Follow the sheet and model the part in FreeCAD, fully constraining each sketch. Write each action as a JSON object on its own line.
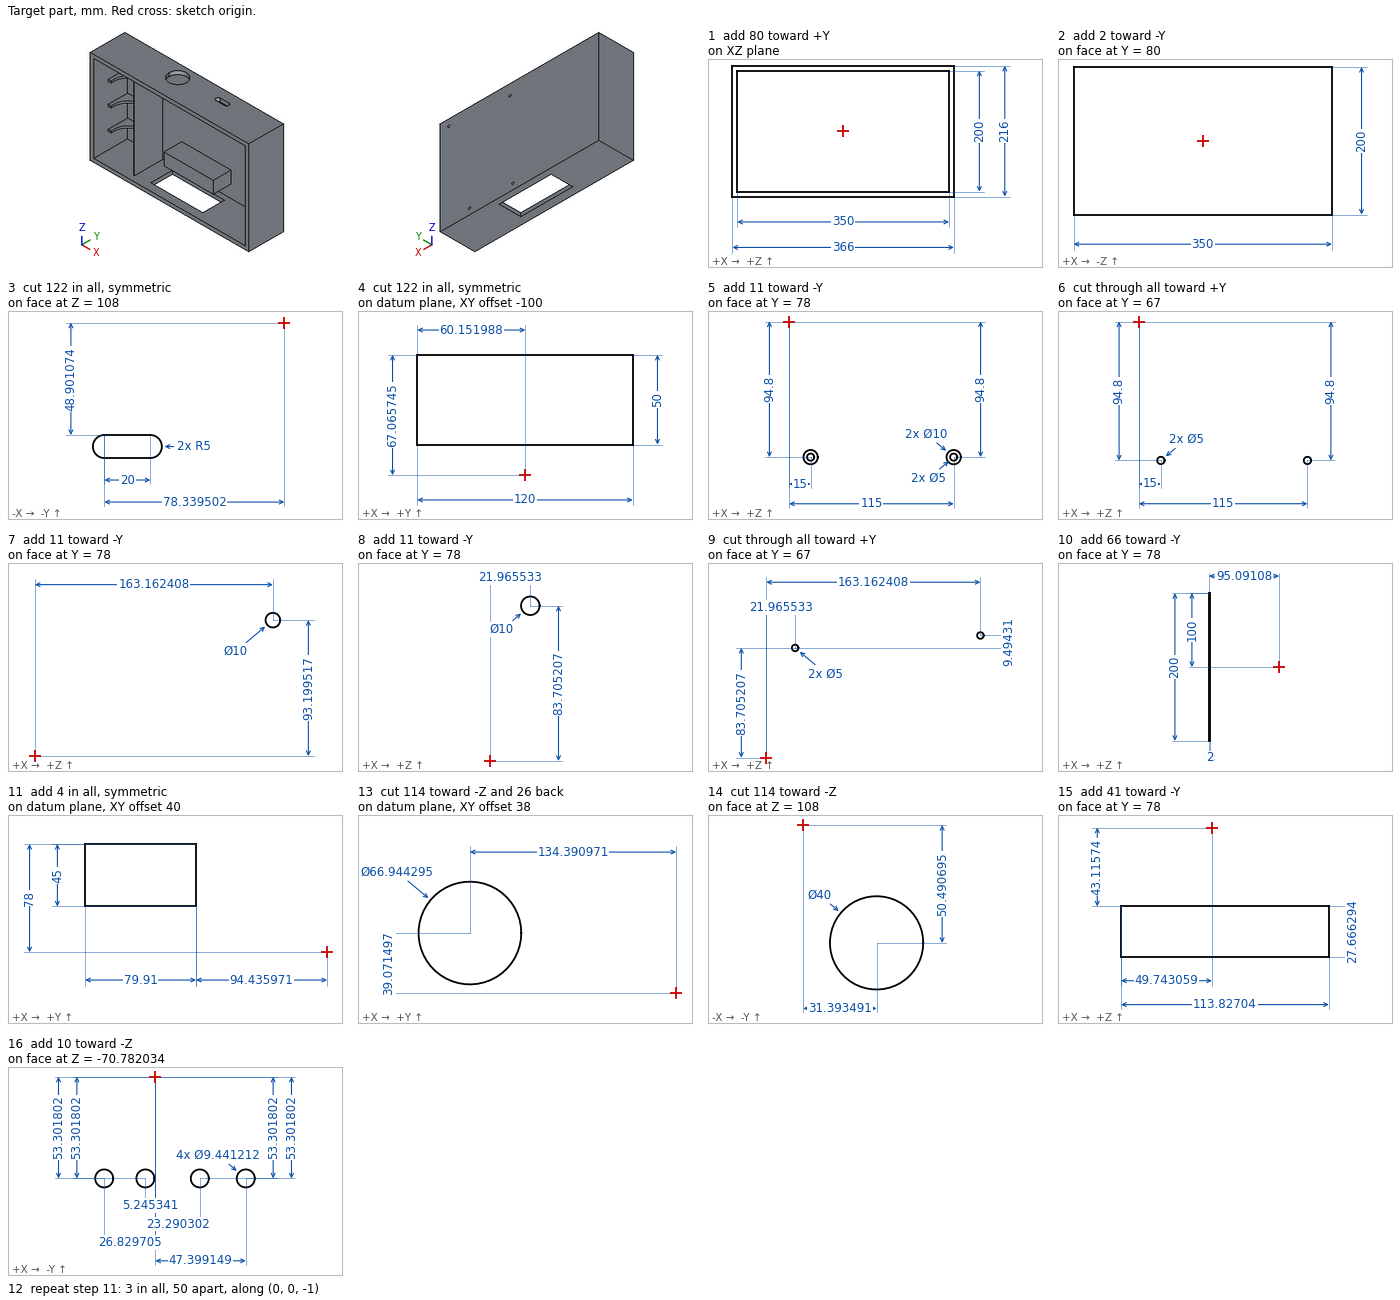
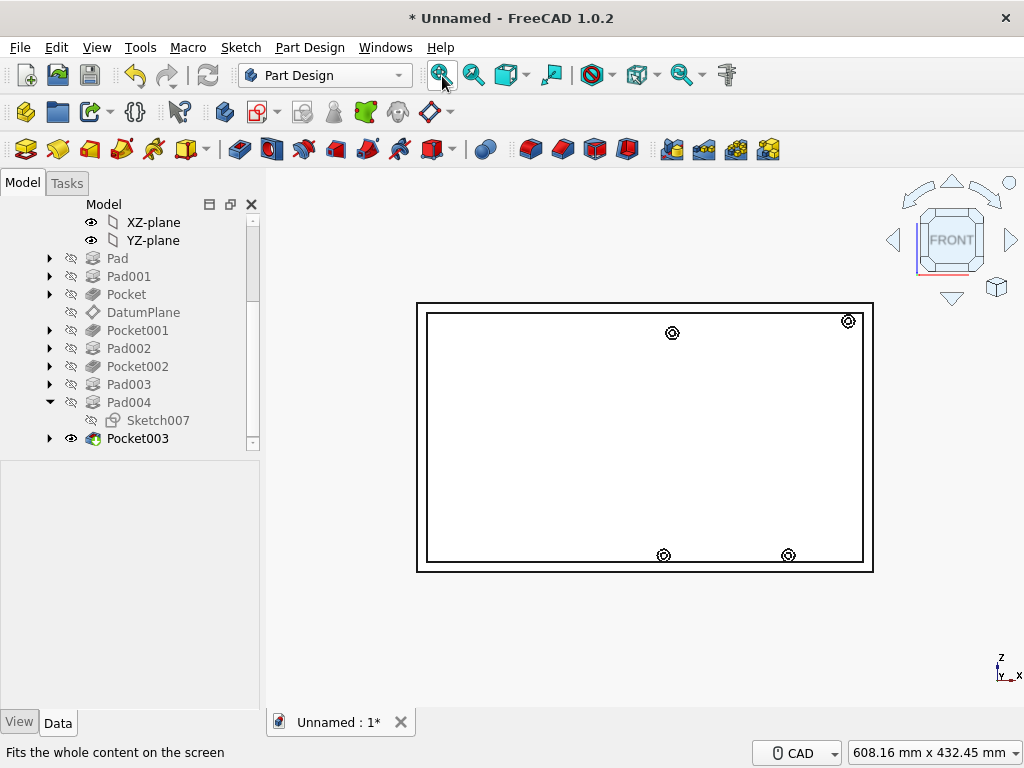
{"action": "left_click", "coordinate": [583, 437]}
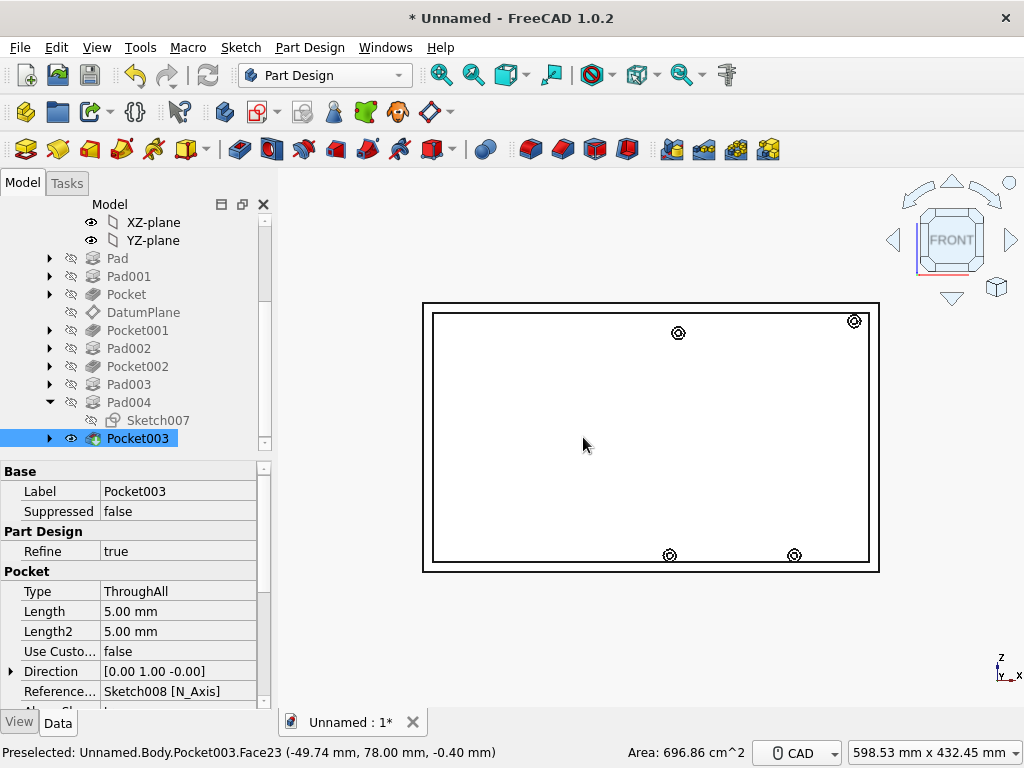
{"action": "left_click", "coordinate": [258, 112]}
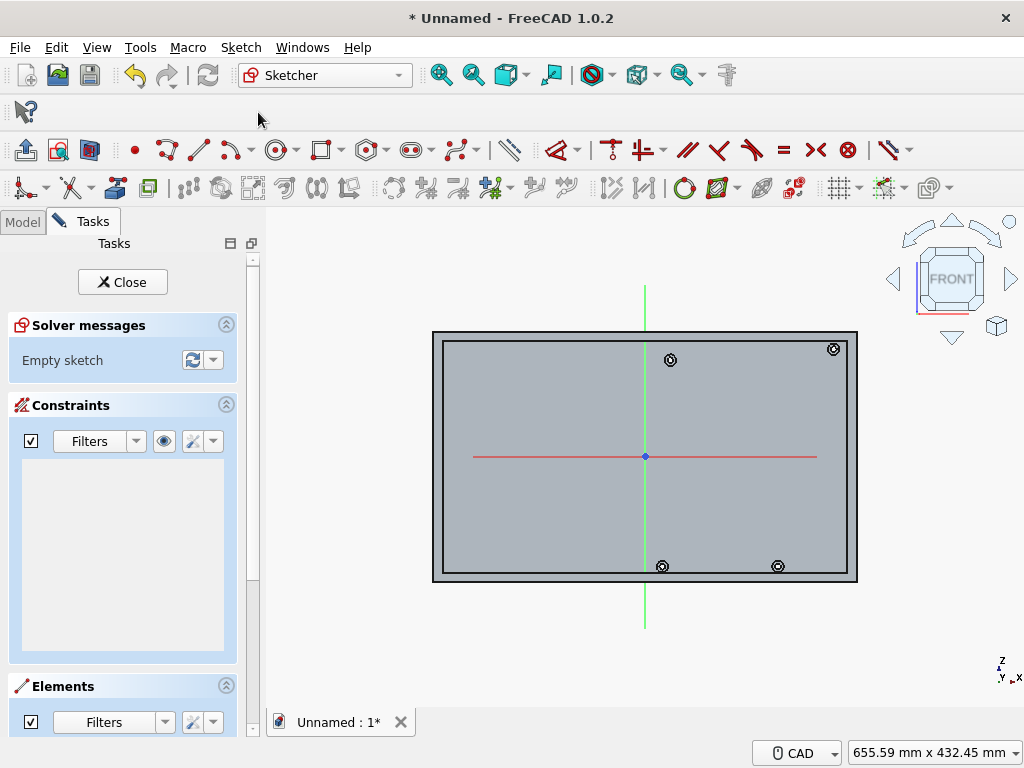
{"action": "scroll", "coordinate": [618, 457], "scroll_direction": "up", "scroll_amount": 2}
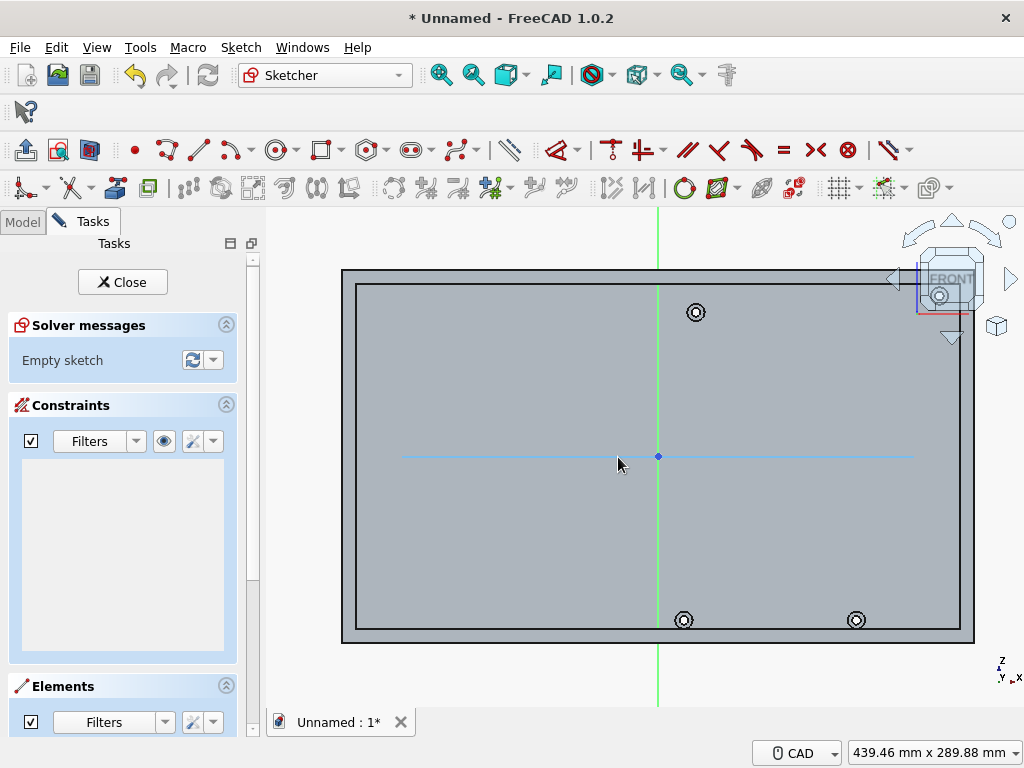
{"action": "key", "text": "g r"}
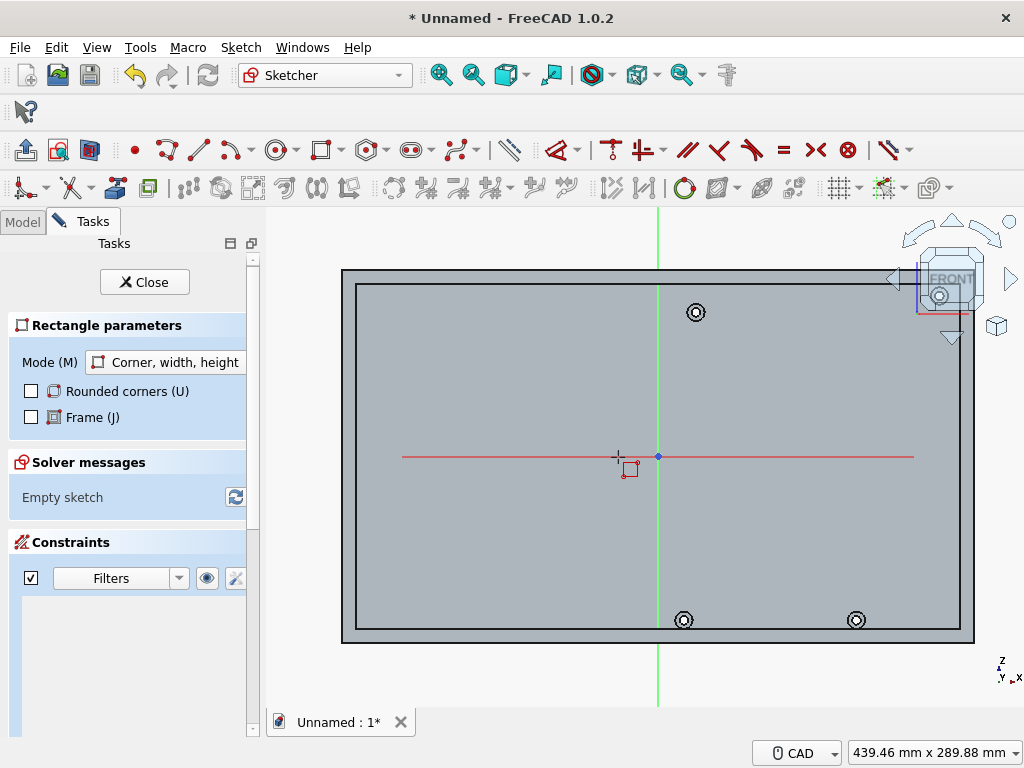
{"action": "scroll", "coordinate": [494, 284], "scroll_direction": "up", "scroll_amount": 8}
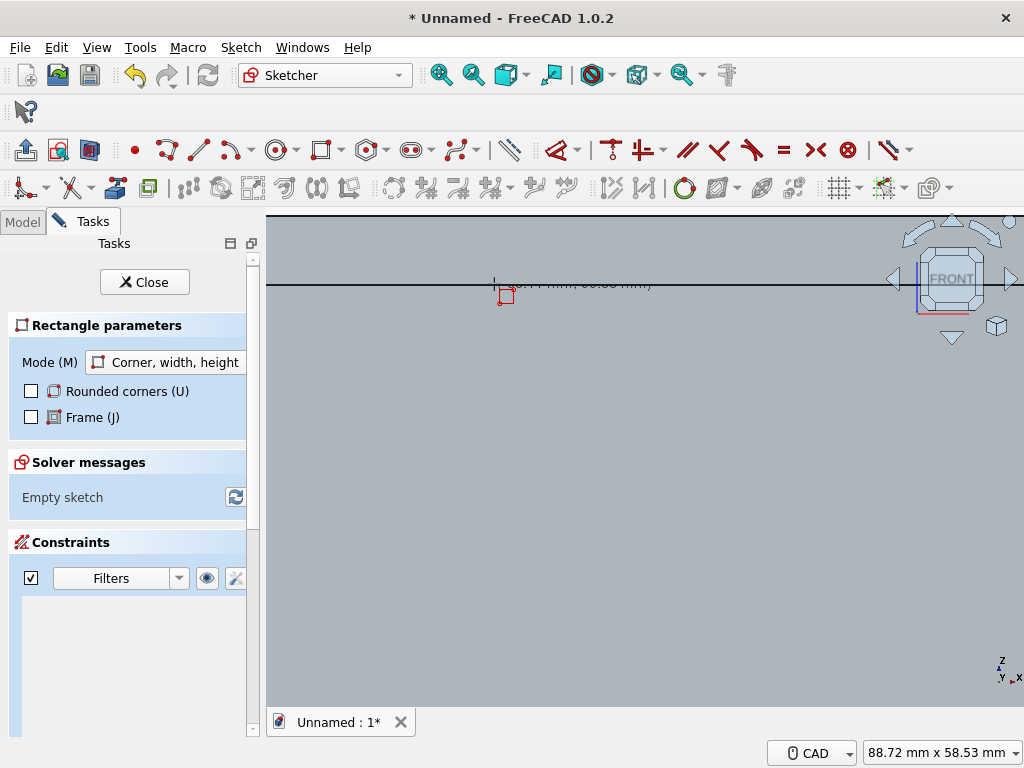
{"action": "scroll", "coordinate": [495, 284], "scroll_direction": "down", "scroll_amount": 8}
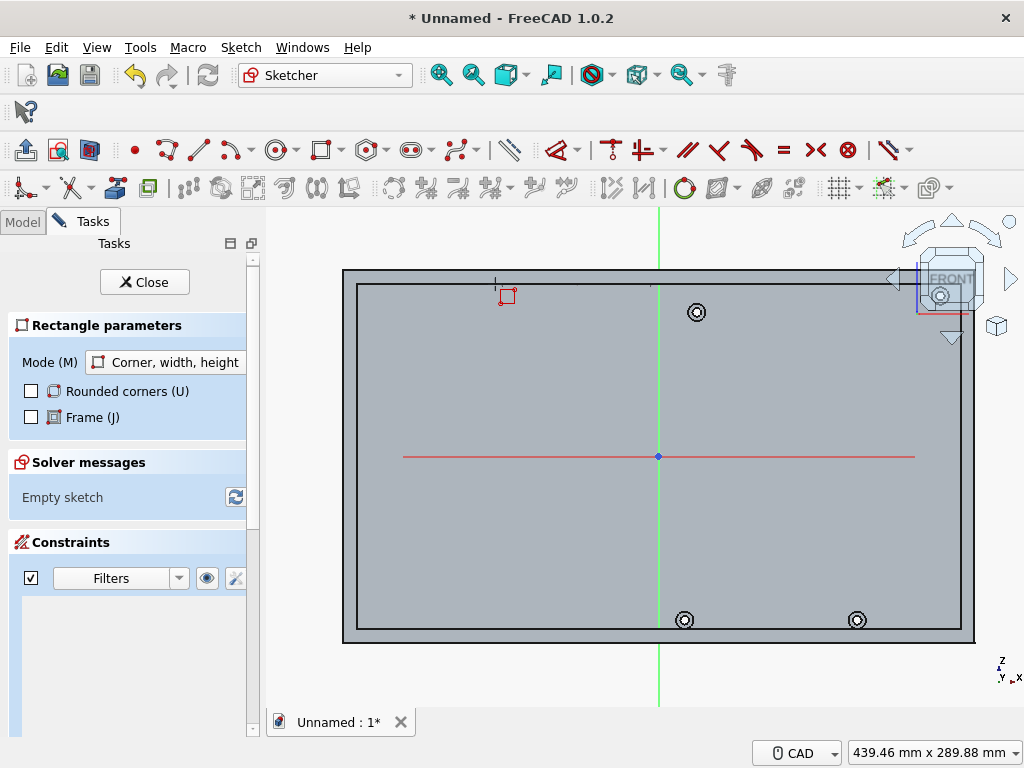
{"action": "left_click", "coordinate": [495, 284]}
{"action": "mouse_move", "coordinate": [498, 629]}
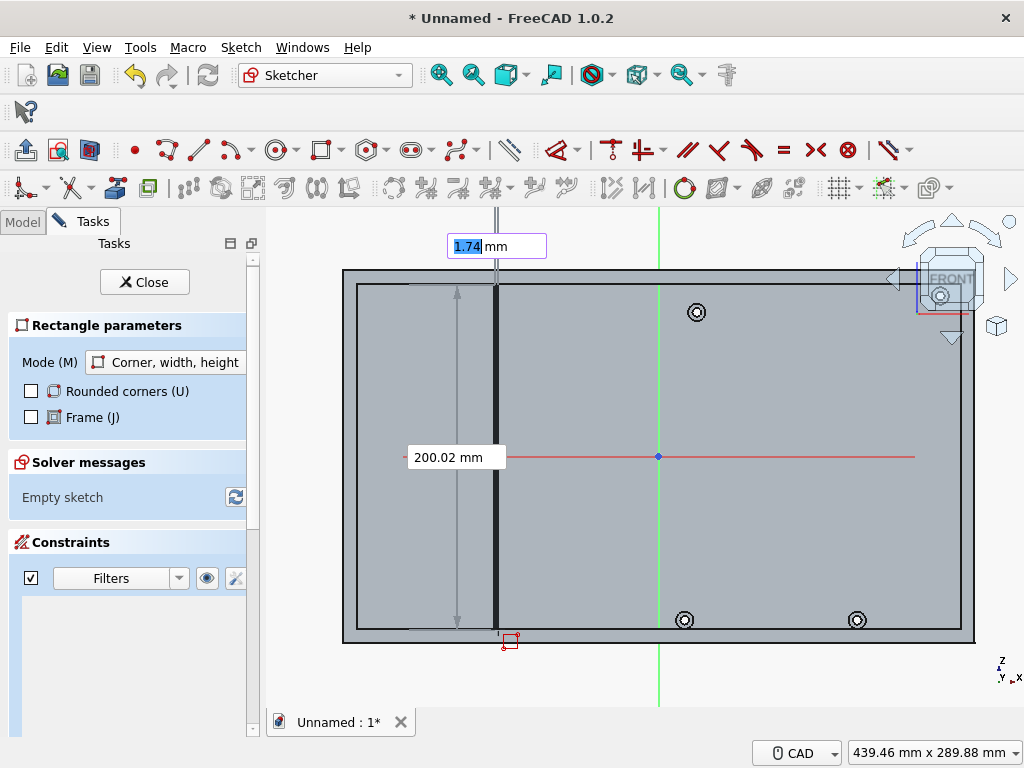
{"action": "type", "text": "2"}
{"action": "key", "text": "Tab"}
{"action": "type", "text": "200"}
{"action": "key", "text": "Return"}
{"action": "key", "text": "Escape"}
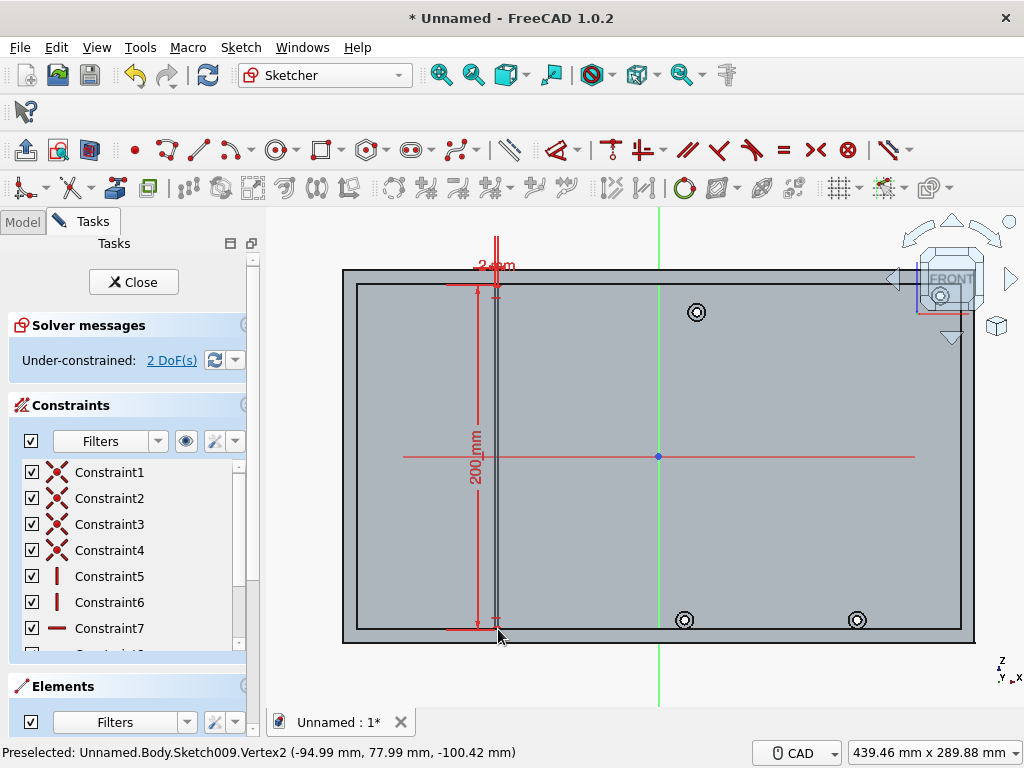
{"action": "left_click", "coordinate": [556, 150]}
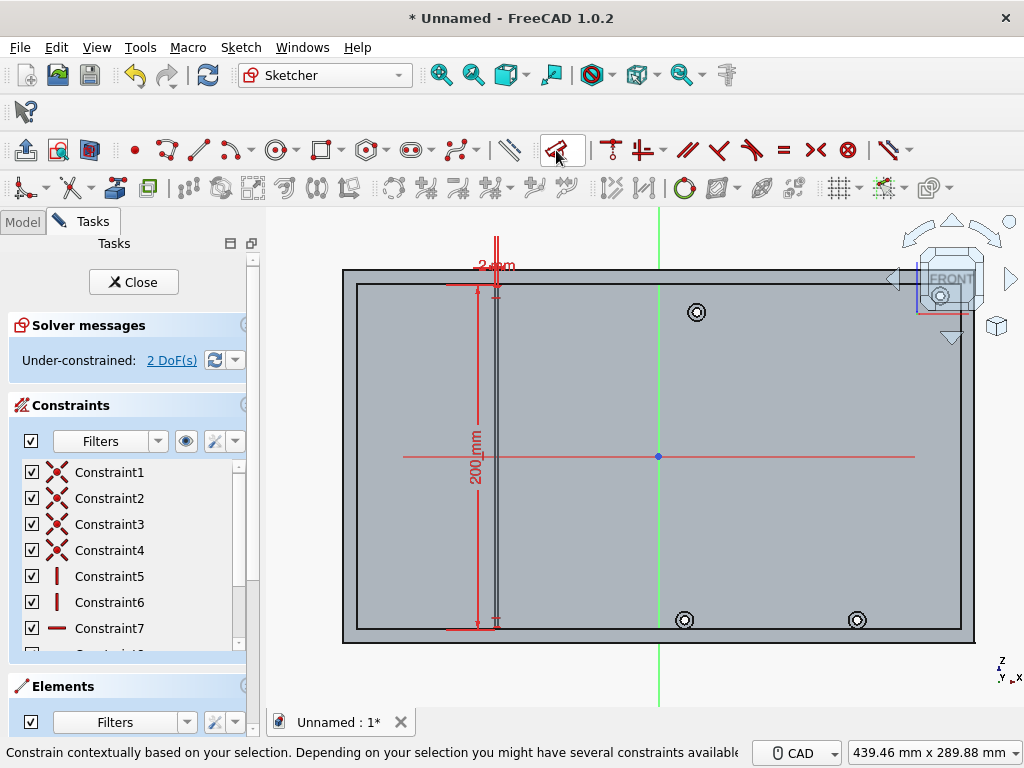
{"action": "scroll", "coordinate": [495, 285], "scroll_direction": "up", "scroll_amount": 7}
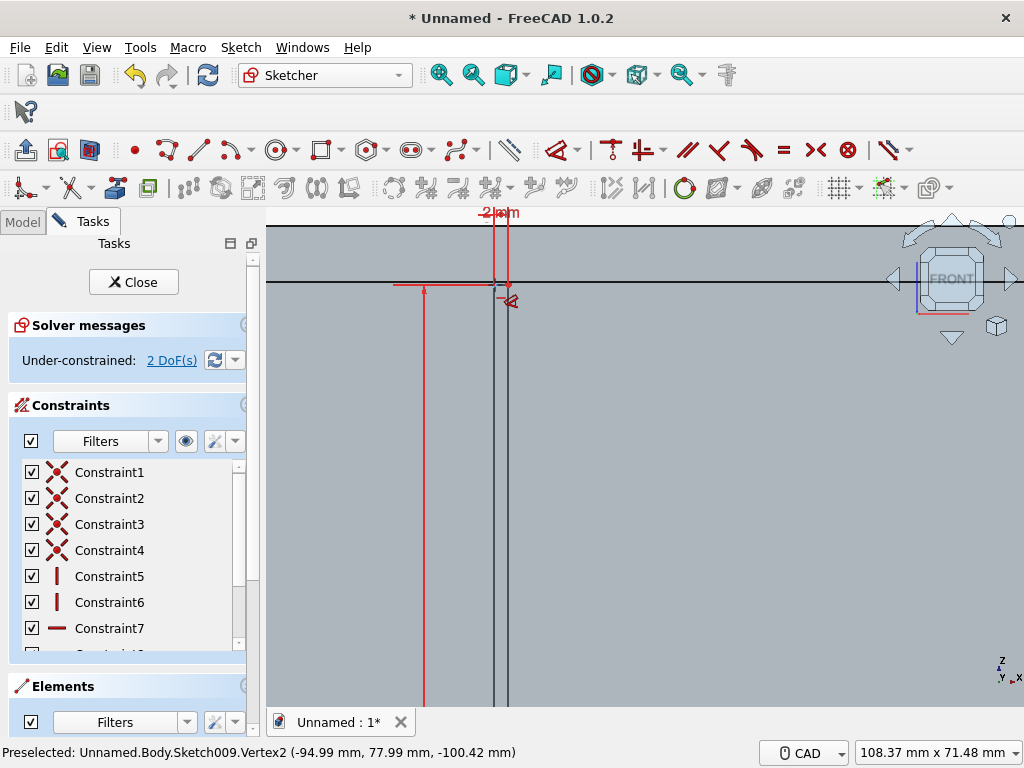
{"action": "left_click", "coordinate": [494, 285]}
{"action": "left_click", "coordinate": [460, 482]}